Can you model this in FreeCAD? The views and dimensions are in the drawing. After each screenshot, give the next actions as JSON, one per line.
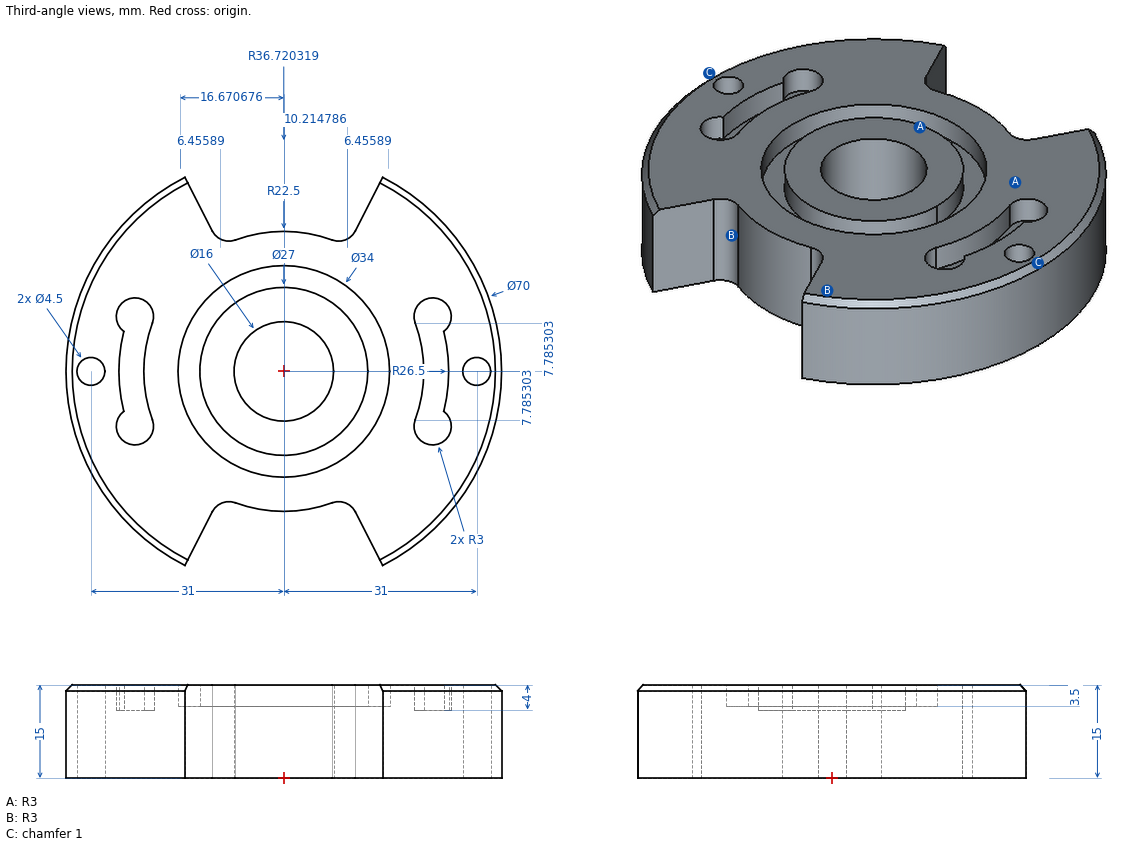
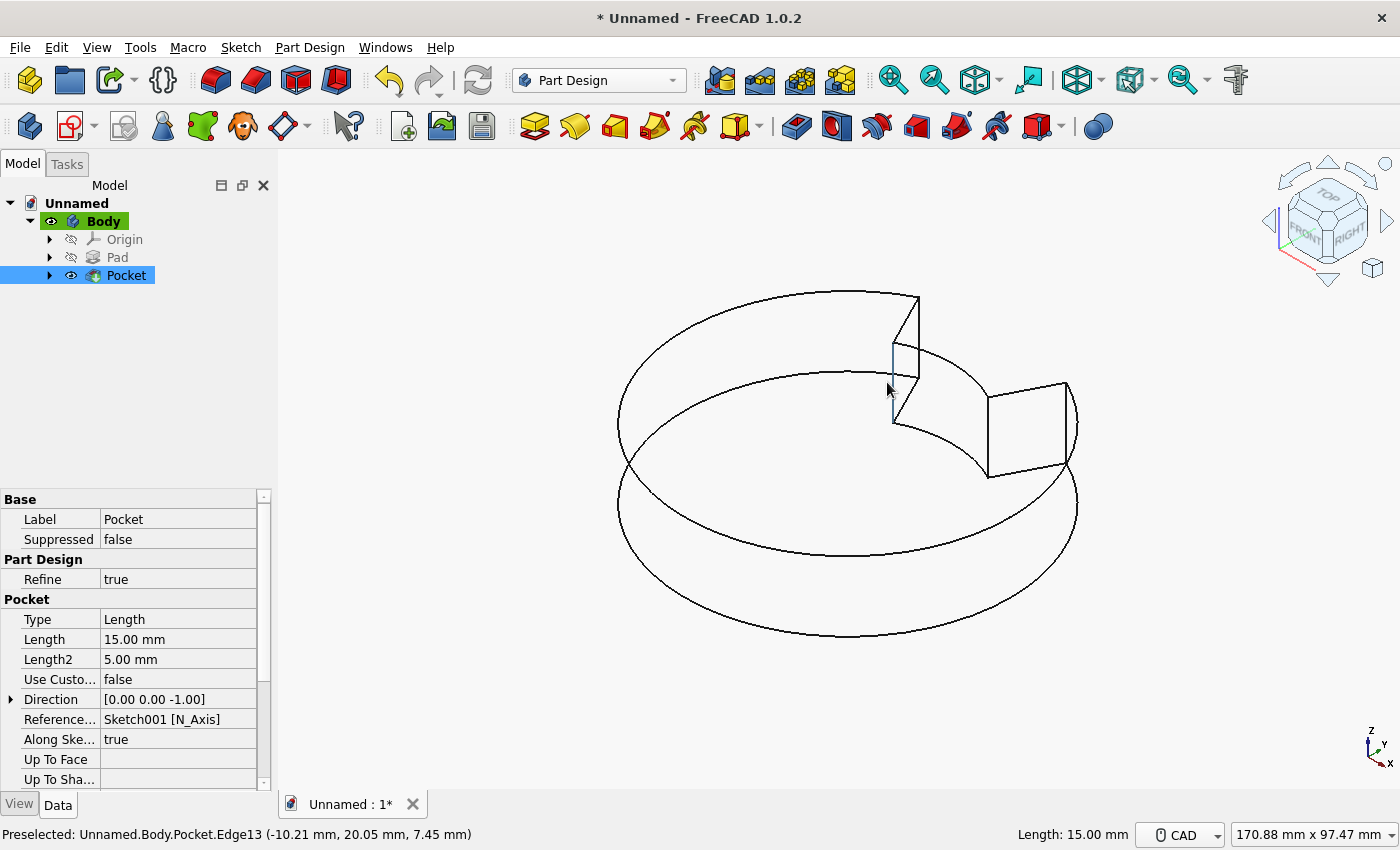
{"action": "left_click", "coordinate": [988, 437], "text": "ctrl"}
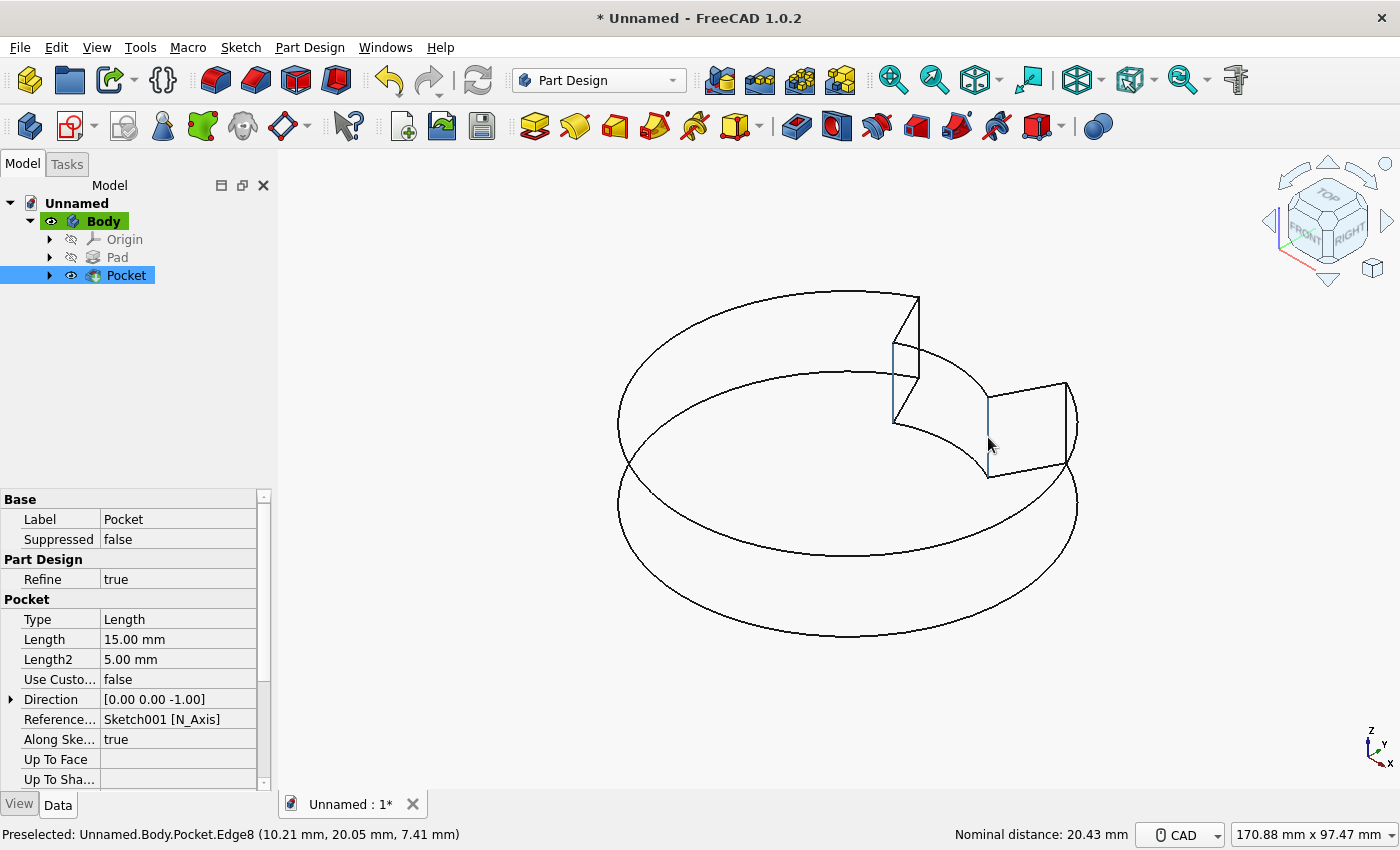
{"action": "key", "text": "v 1"}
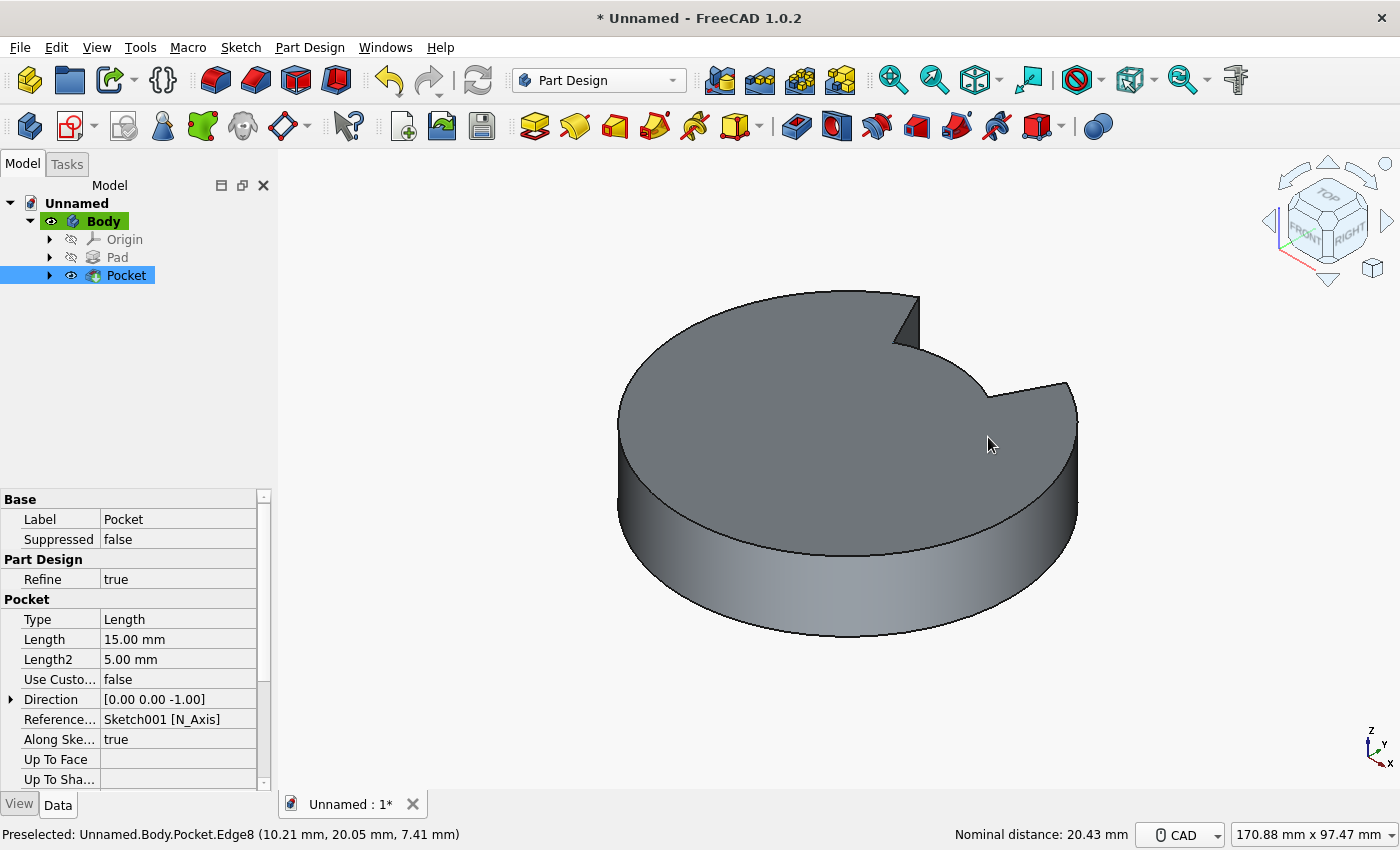
{"action": "left_click", "coordinate": [216, 80]}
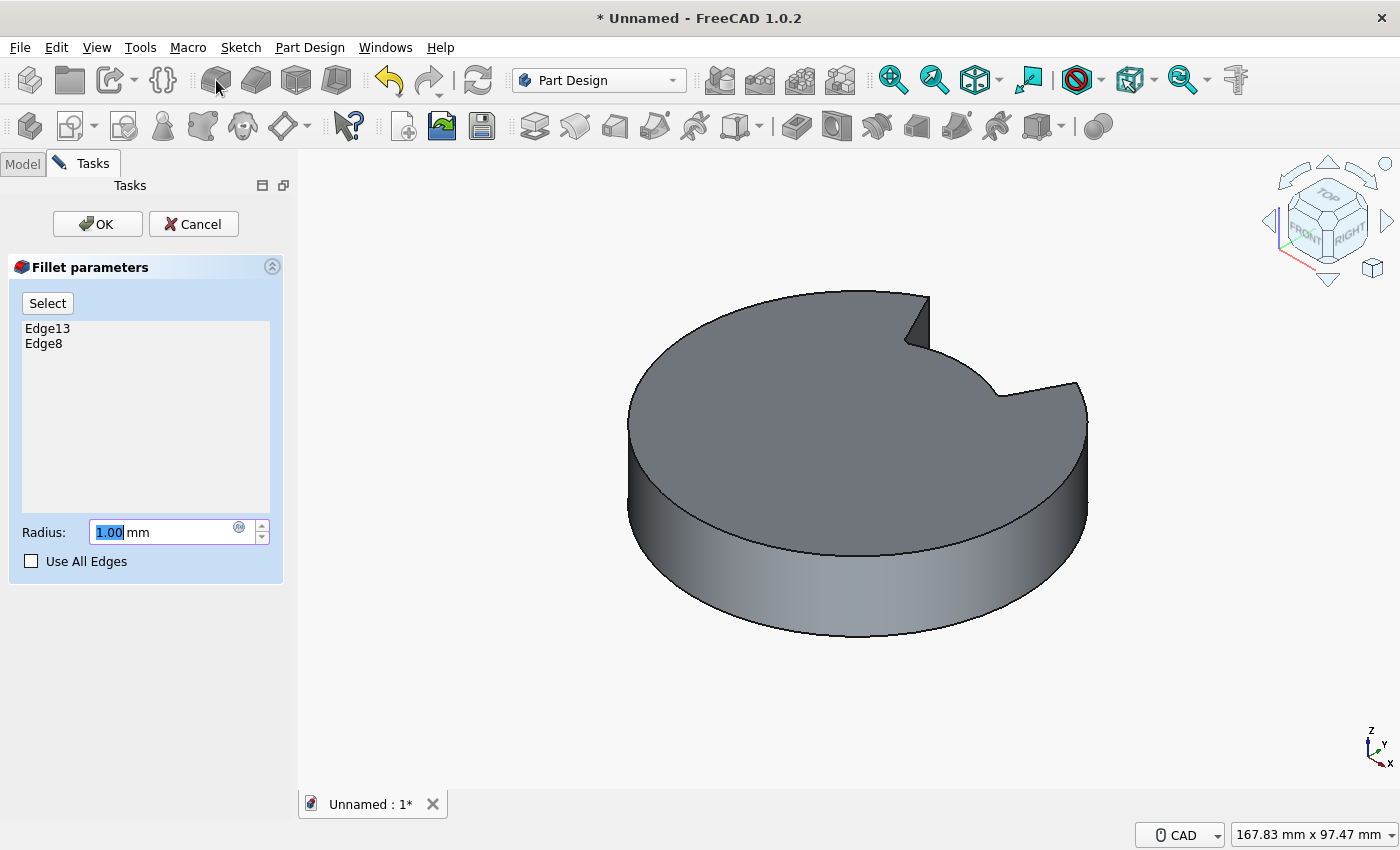
{"action": "type", "text": "3"}
{"action": "key", "text": "Tab"}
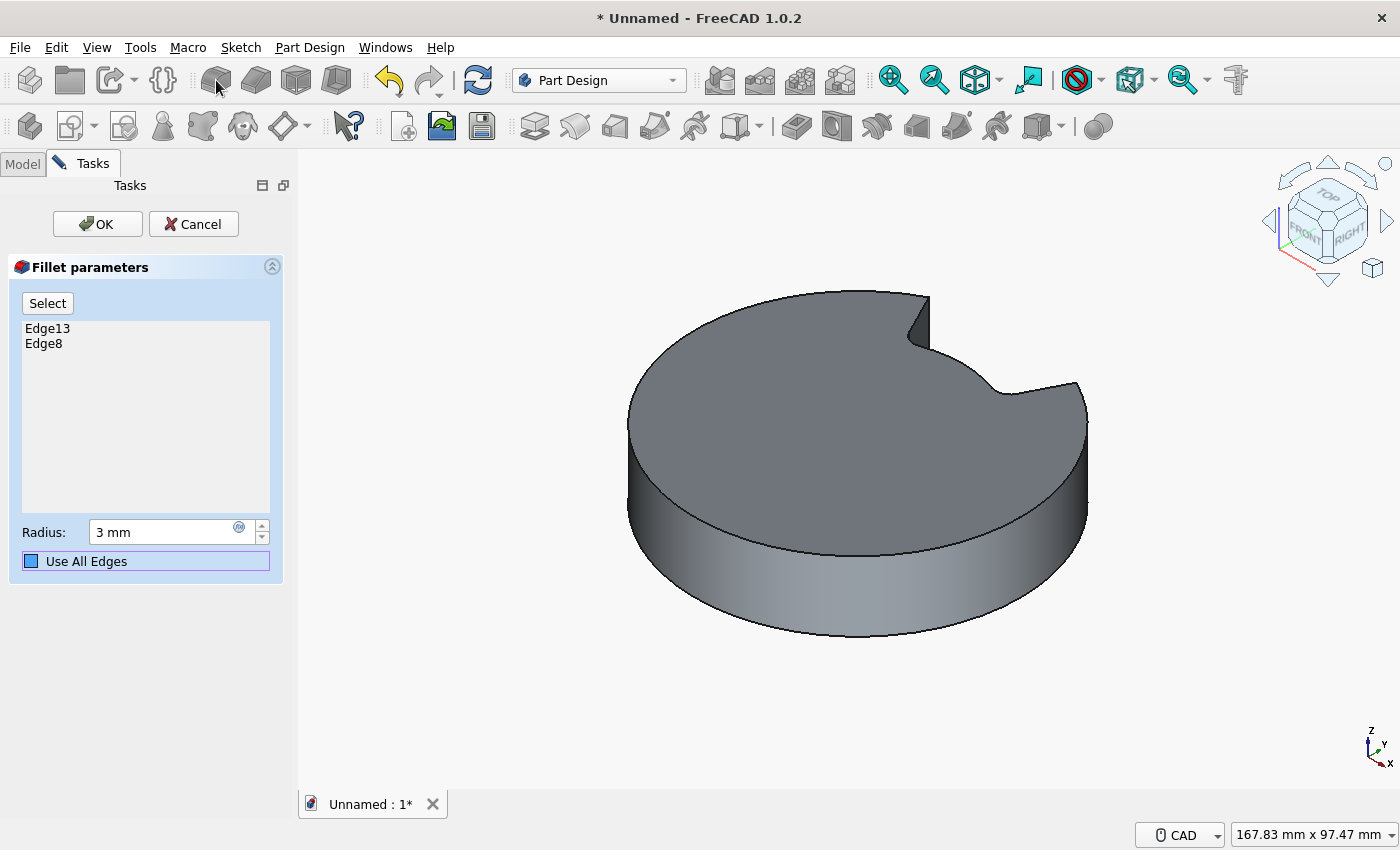
{"action": "left_click", "coordinate": [98, 224]}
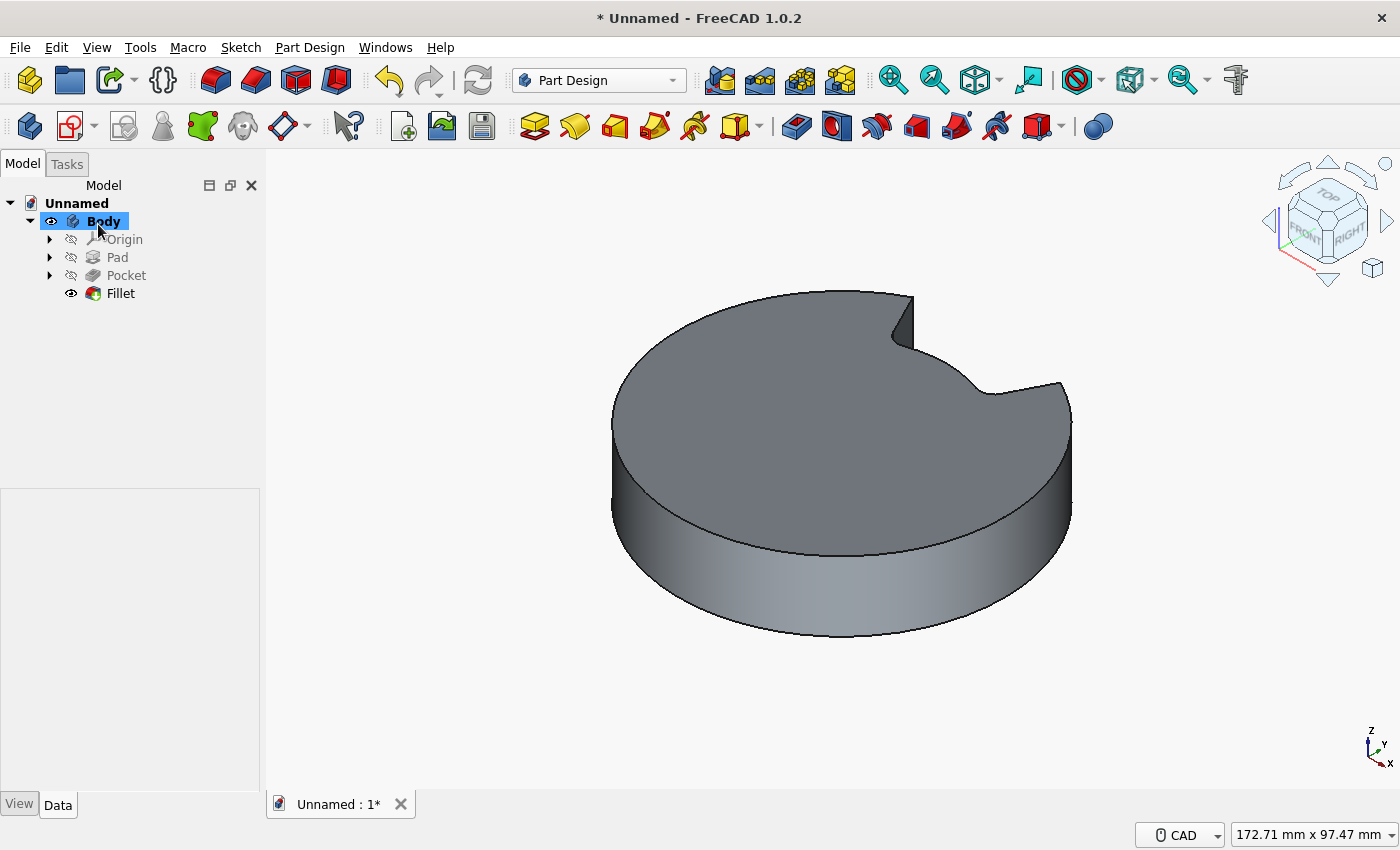
{"action": "left_click", "coordinate": [116, 275]}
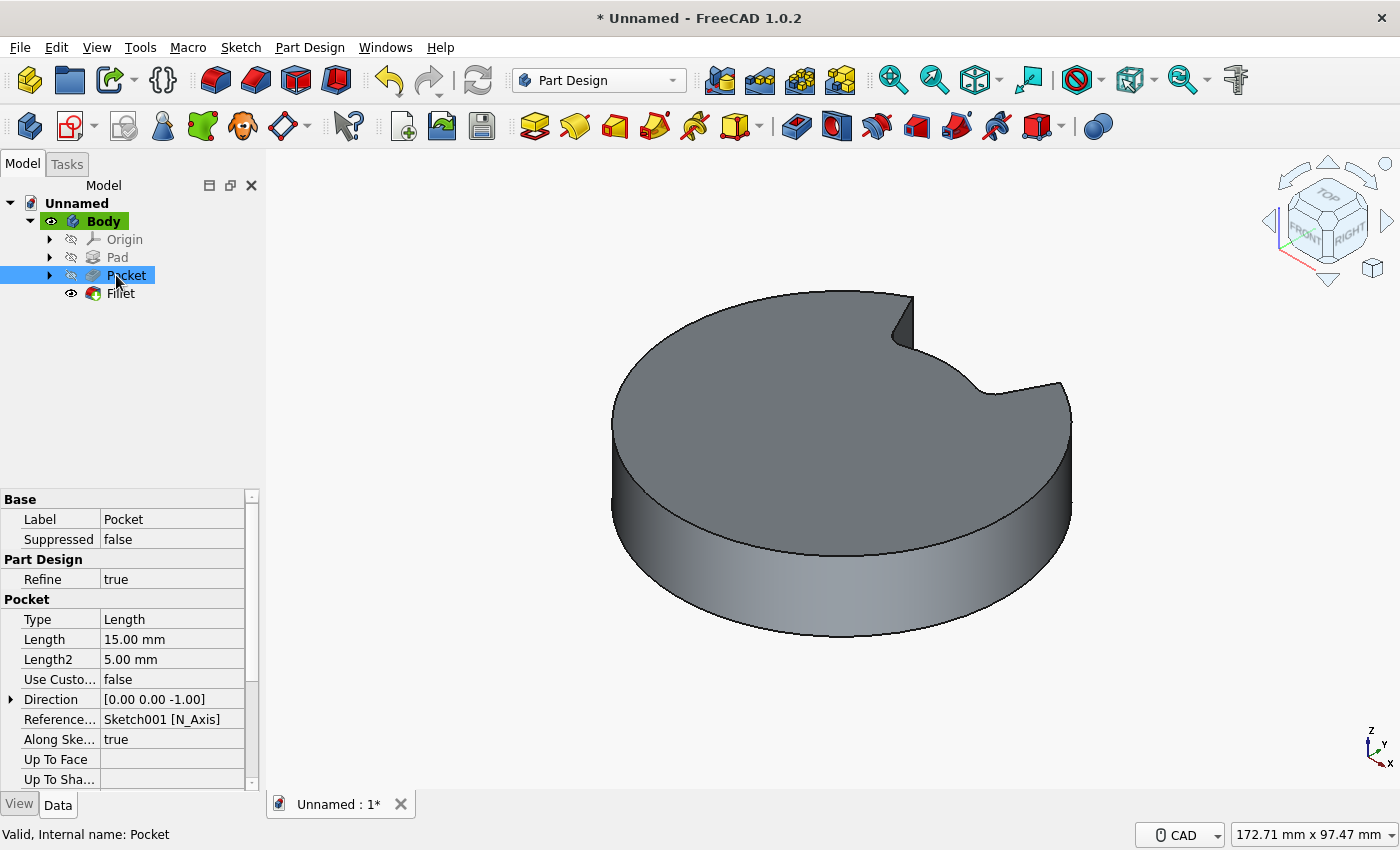
{"action": "left_click", "coordinate": [720, 80]}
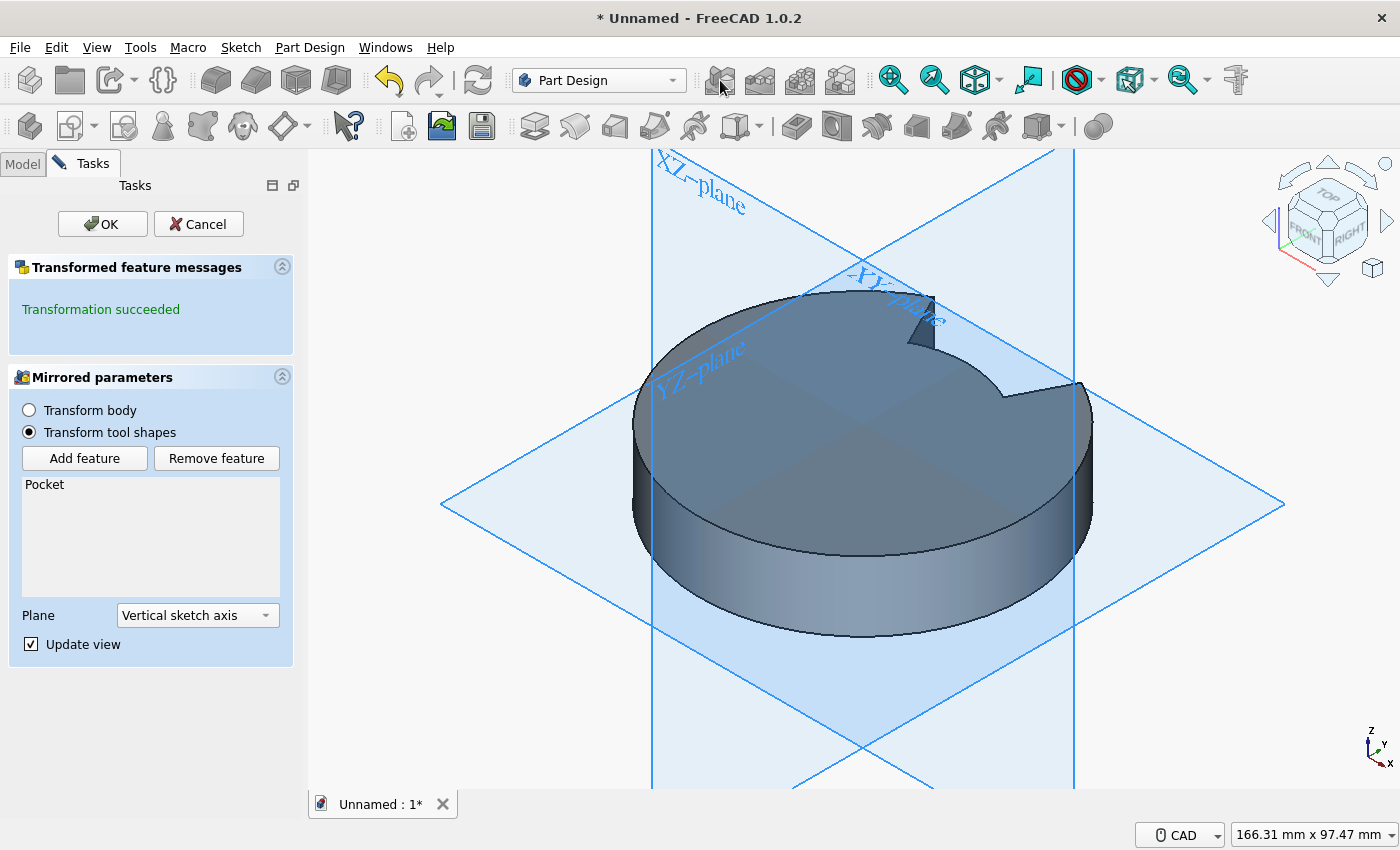
{"action": "left_click", "coordinate": [198, 616]}